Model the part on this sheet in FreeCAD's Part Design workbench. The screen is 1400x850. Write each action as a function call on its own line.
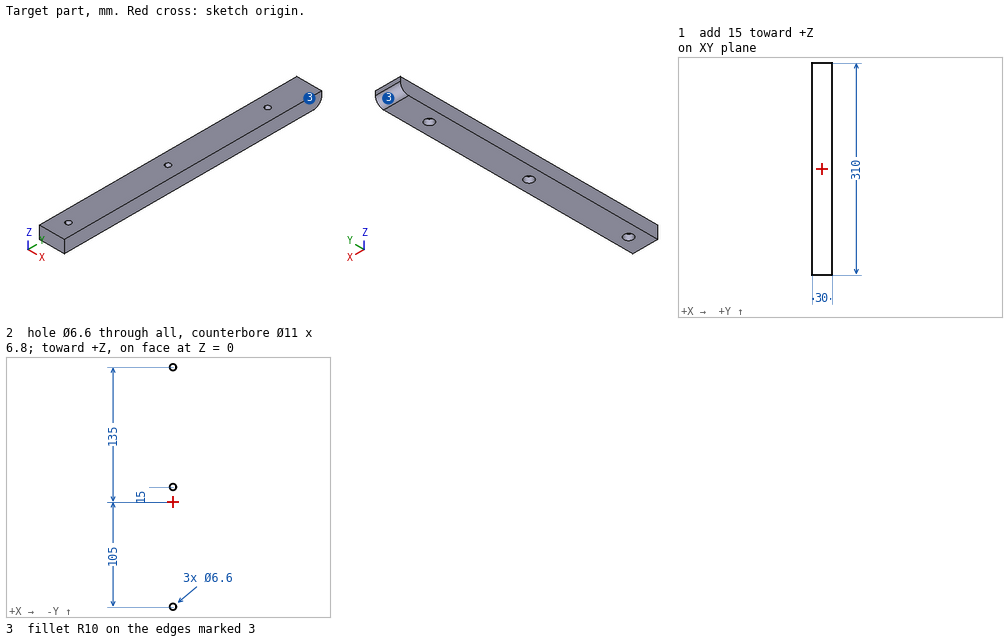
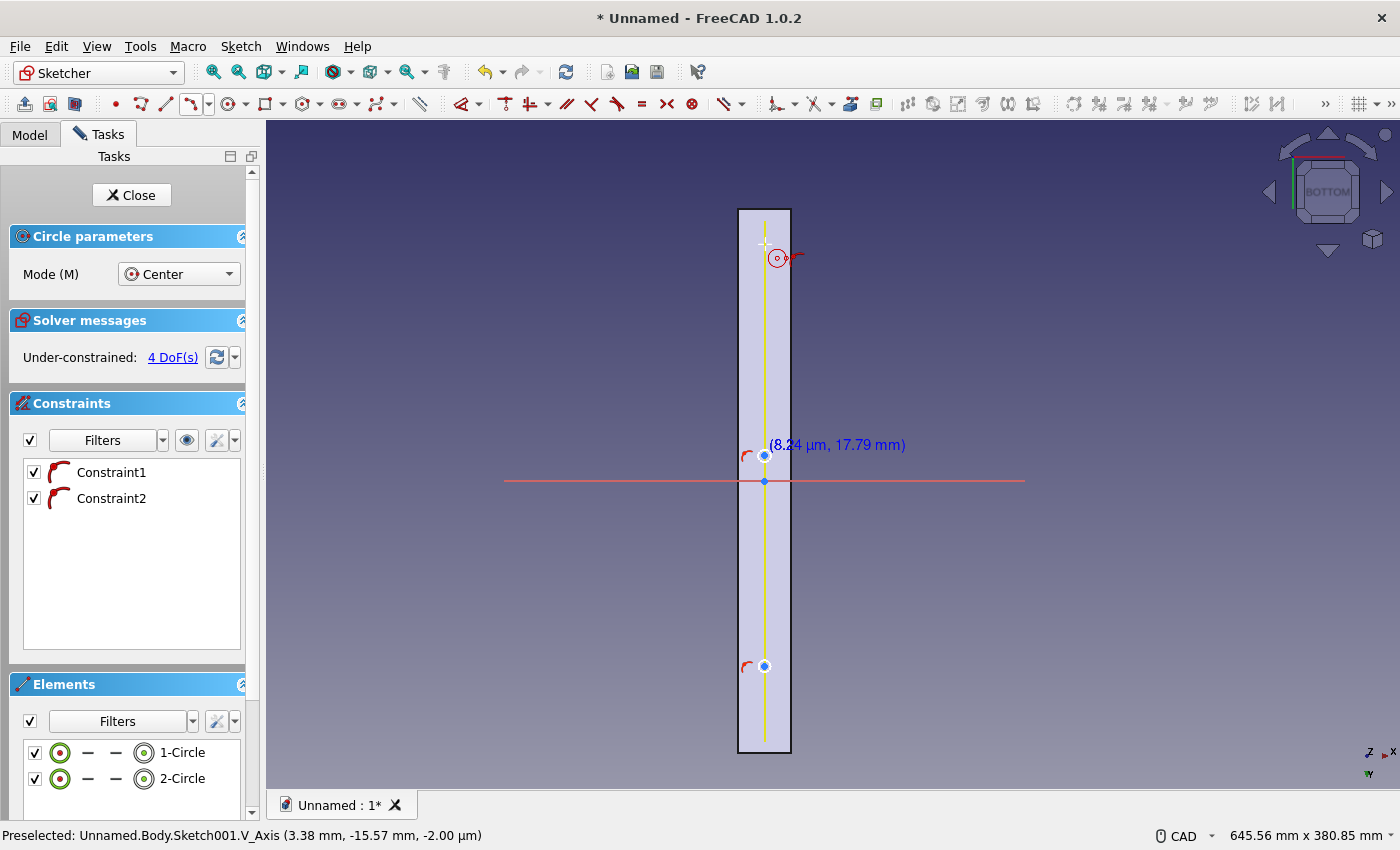
click(765, 244)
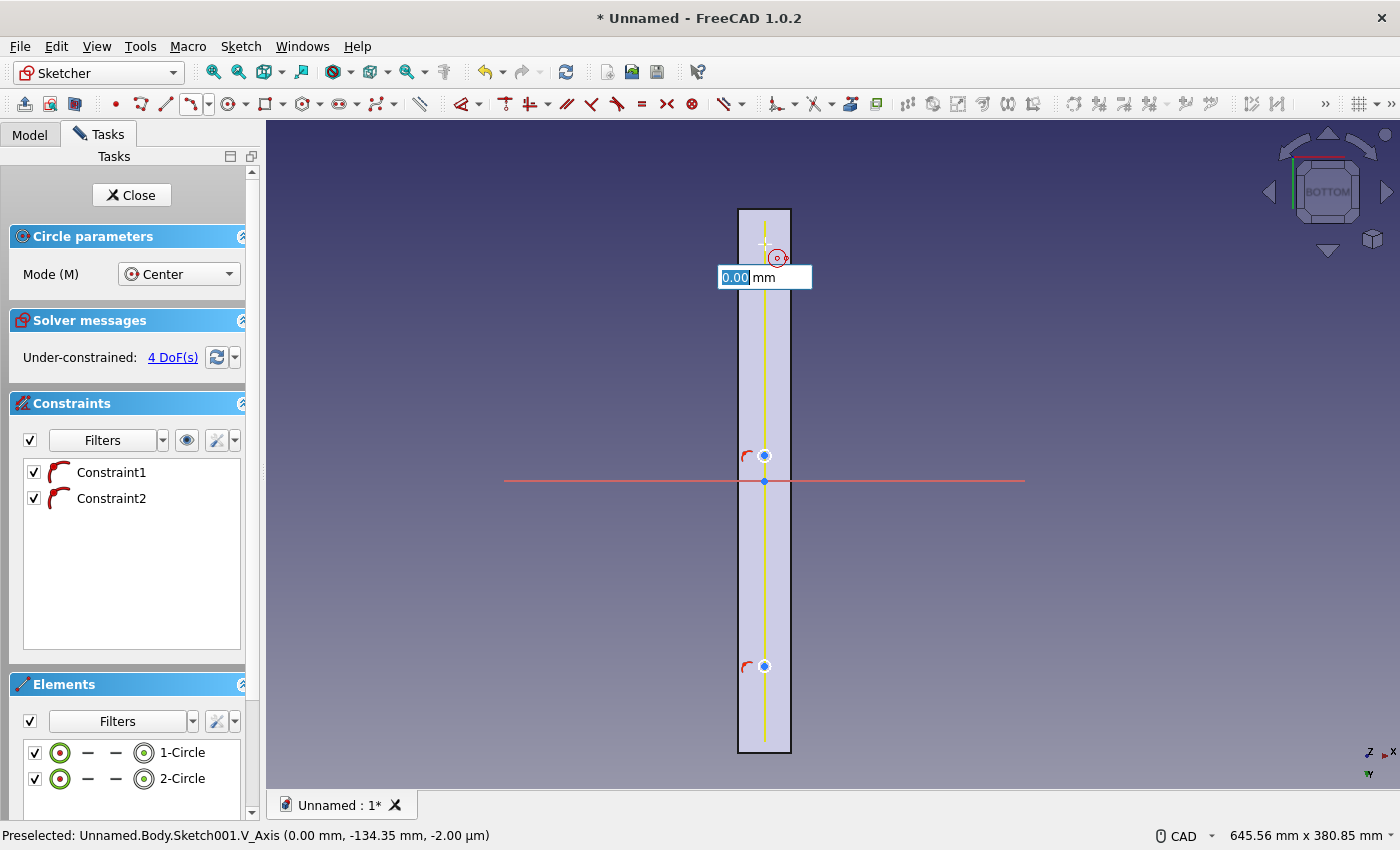
scroll(770, 242, up, 6)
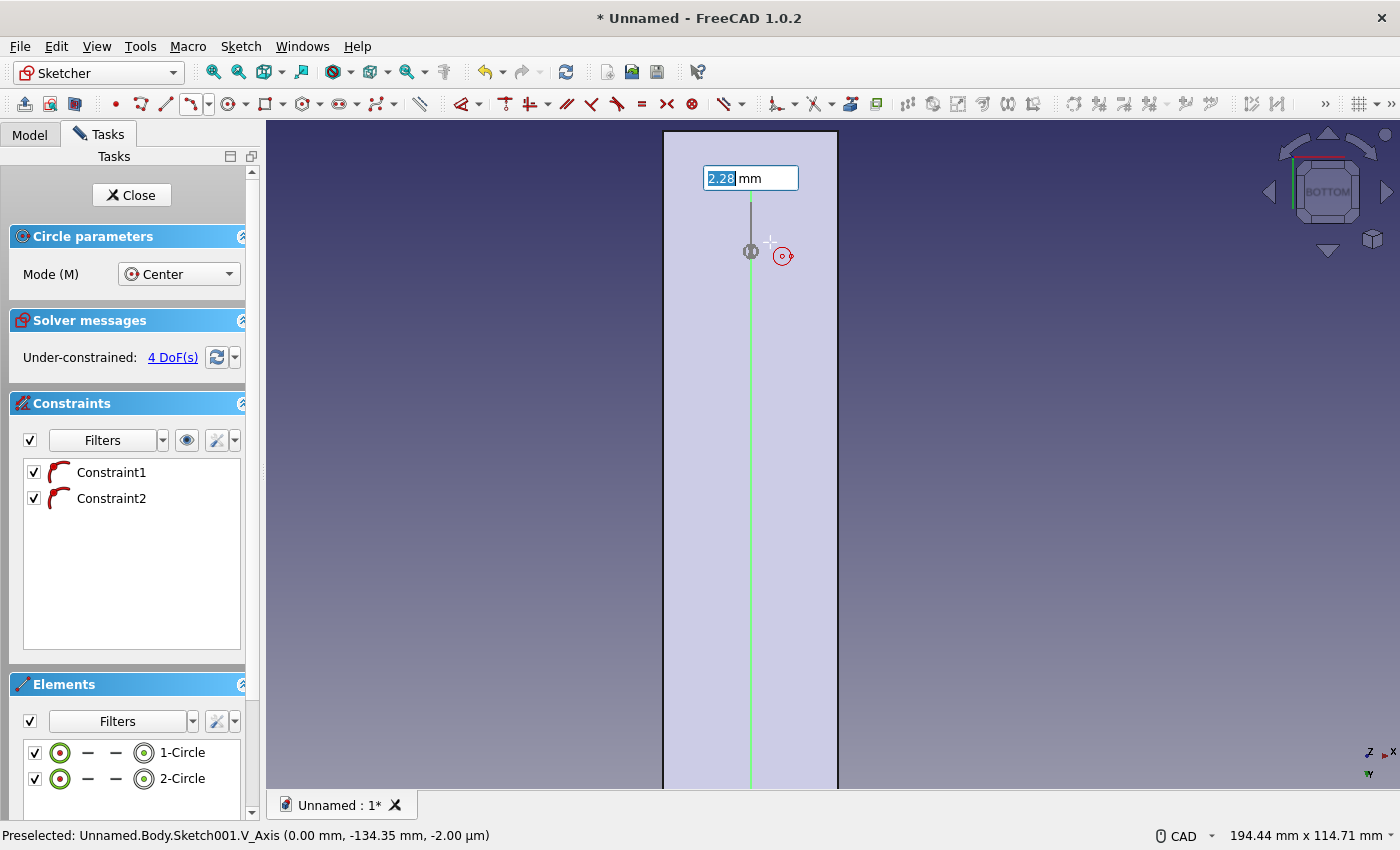
click(769, 241)
key(Escape)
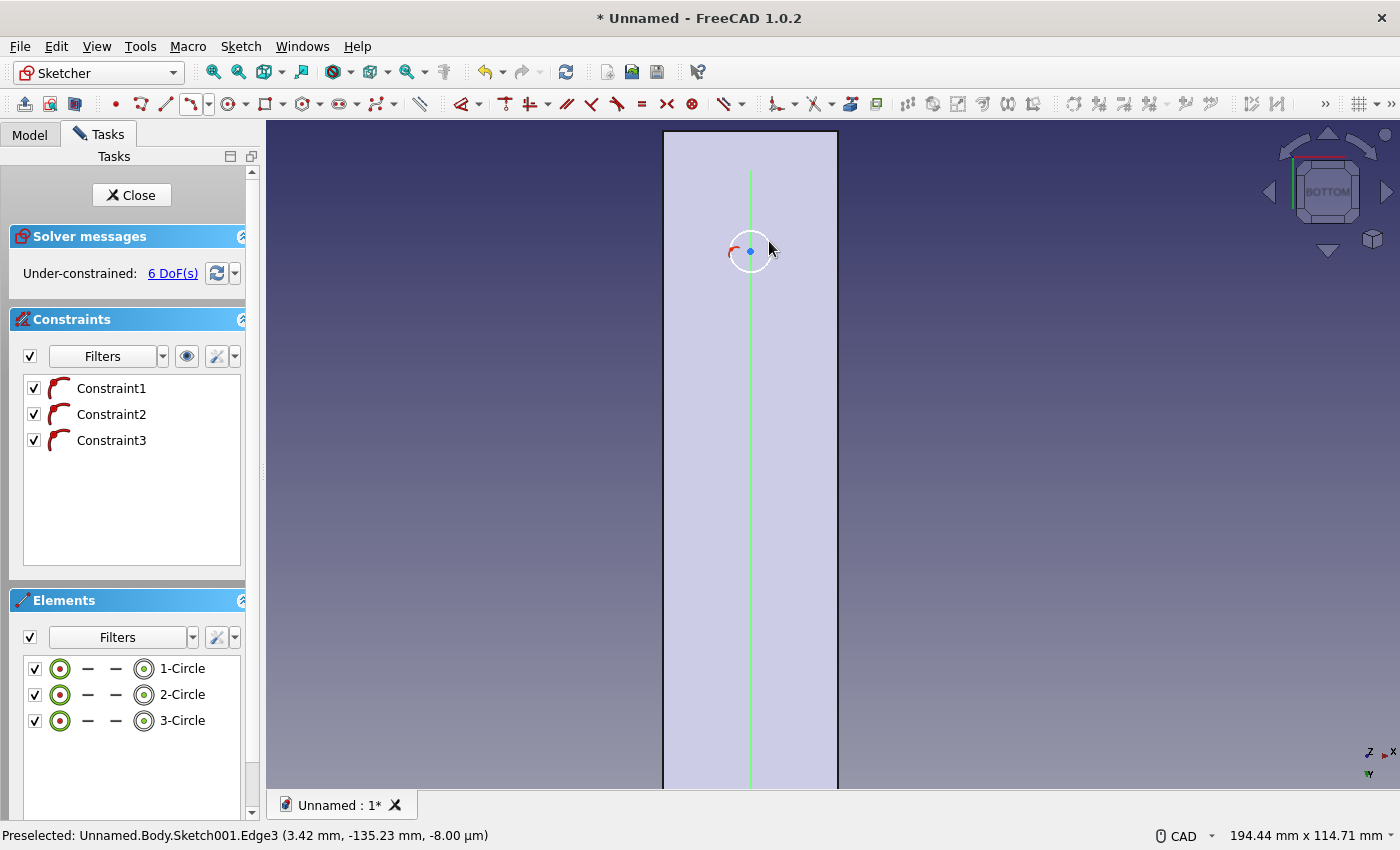
scroll(770, 242, down, 6)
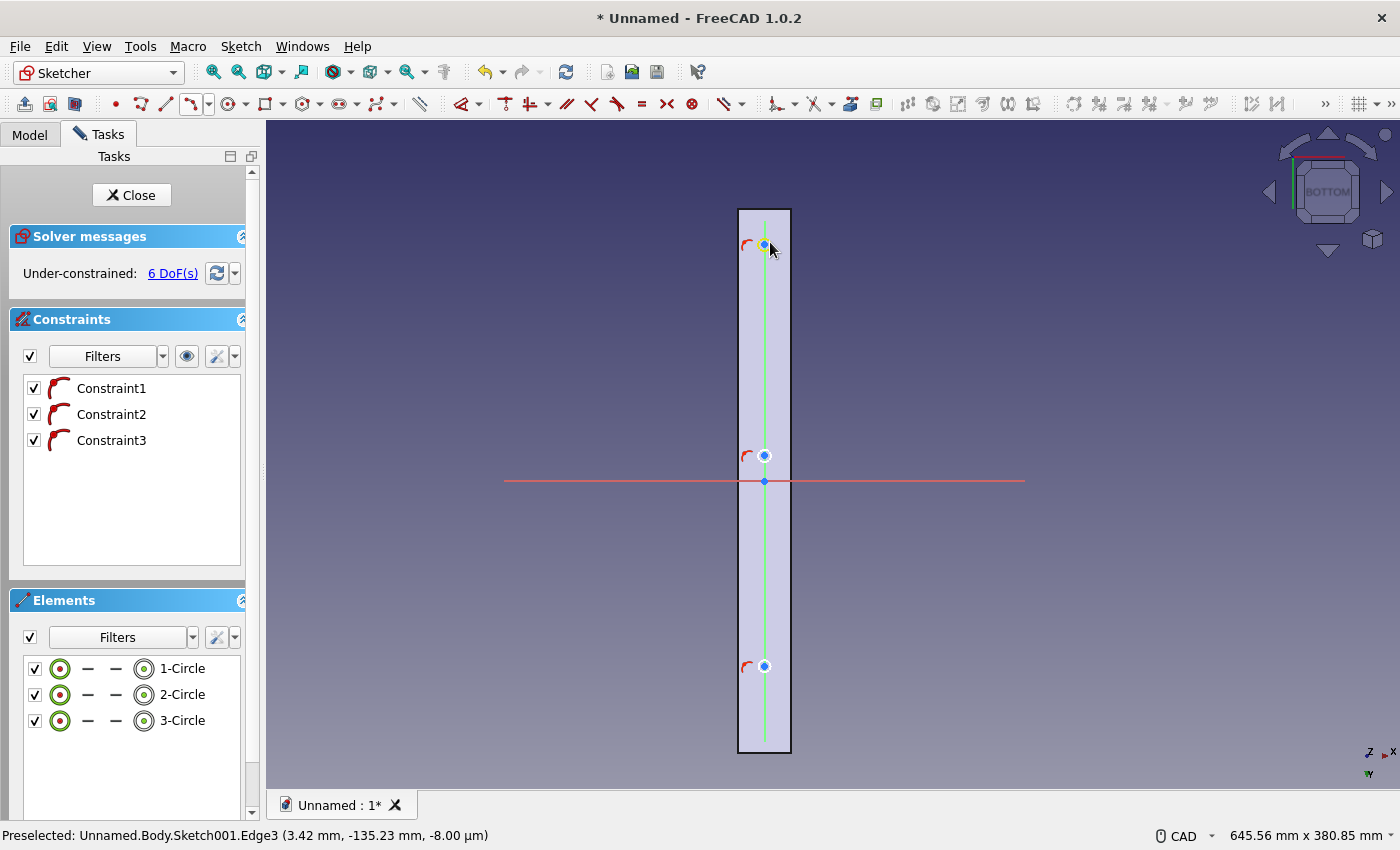
scroll(769, 662, up, 6)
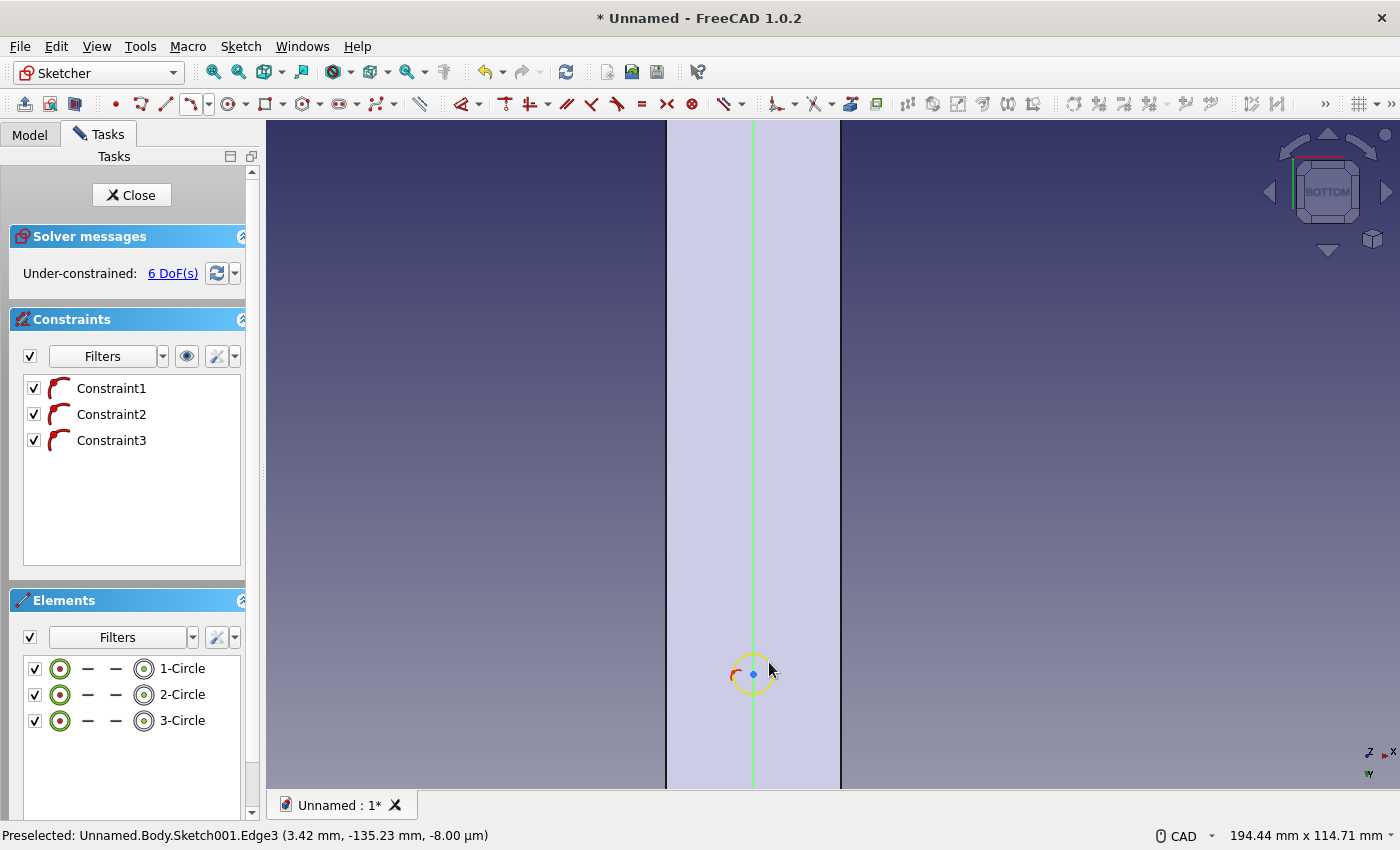
click(767, 660)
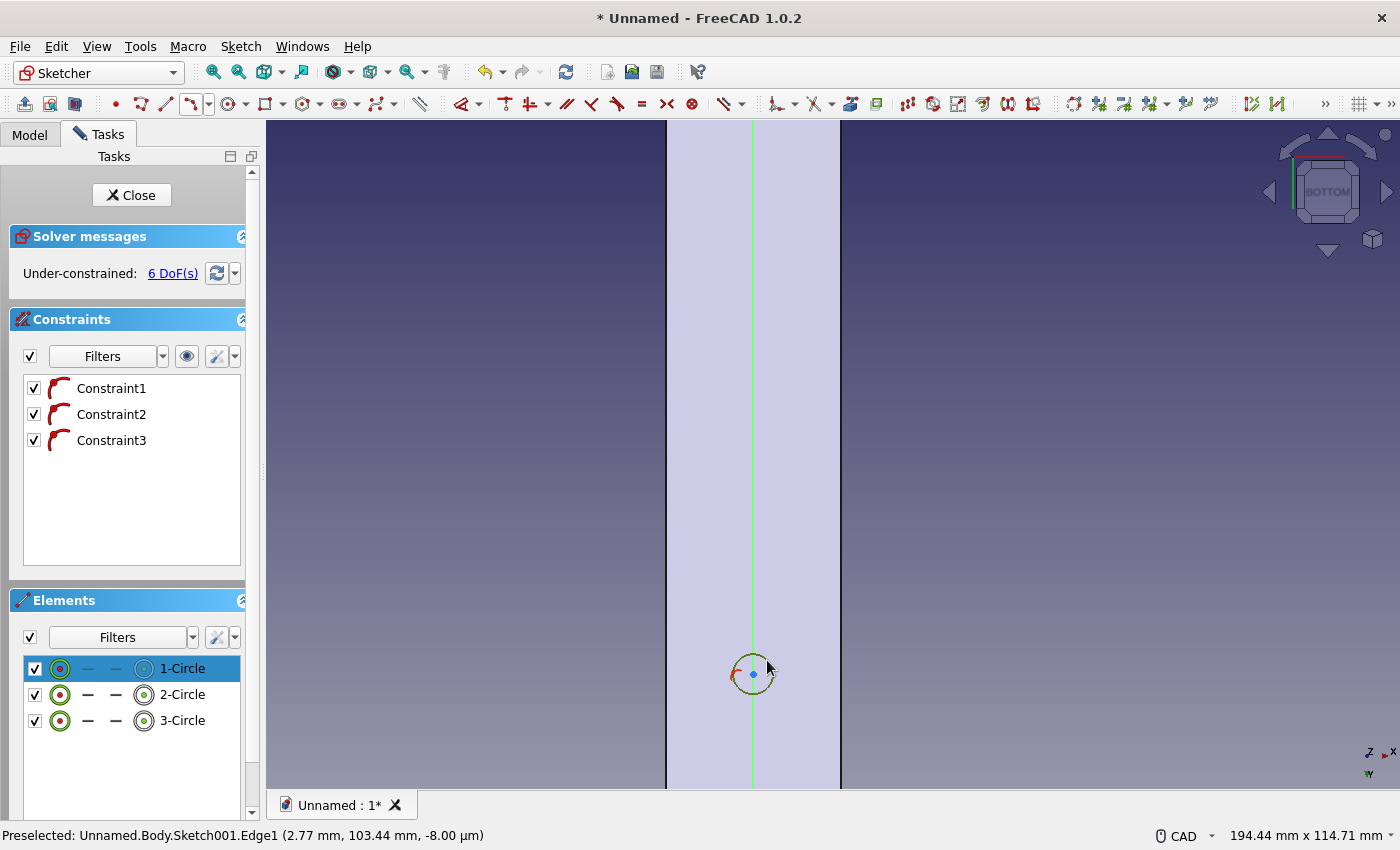
scroll(769, 663, down, 6)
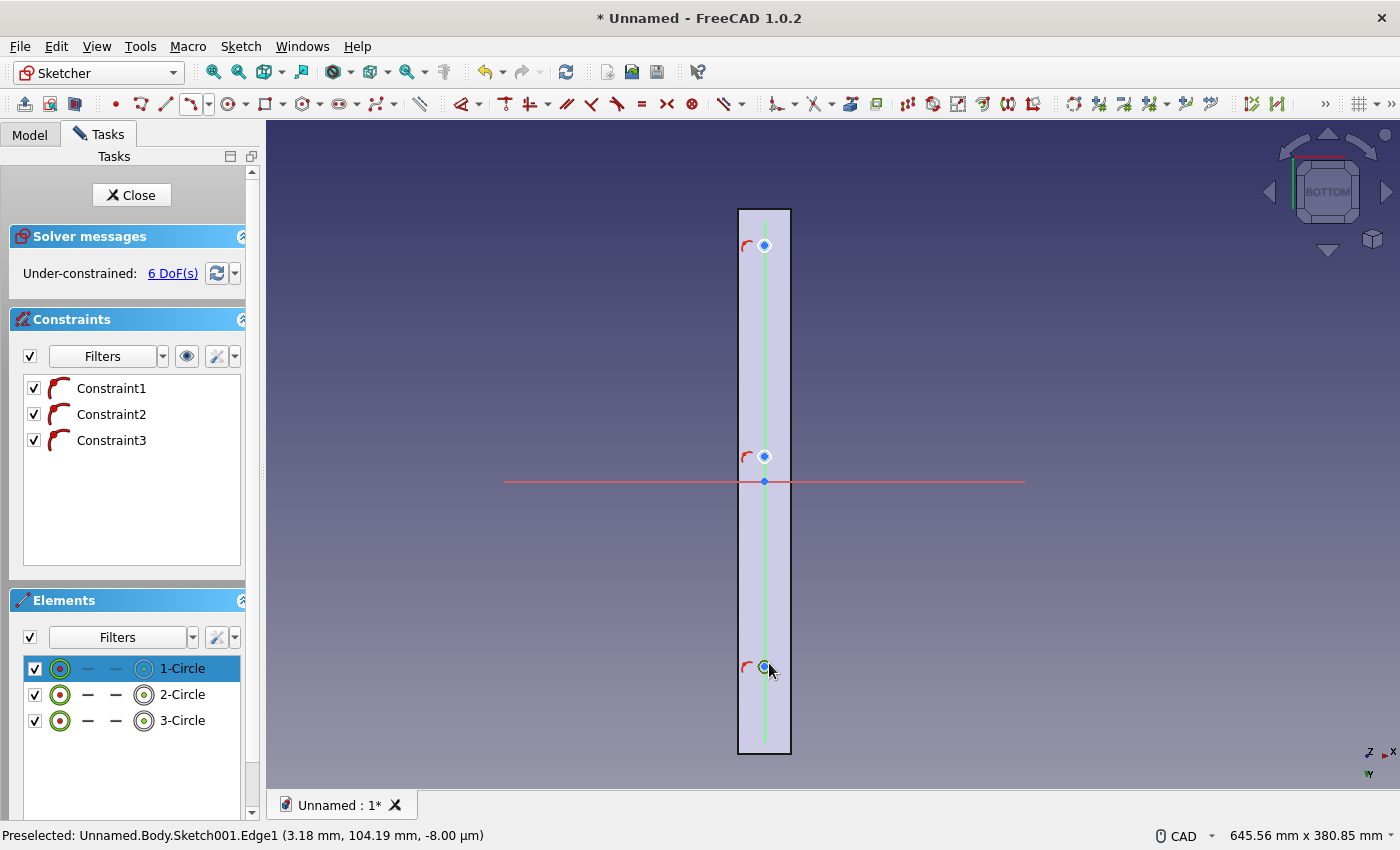
scroll(769, 452, up, 6)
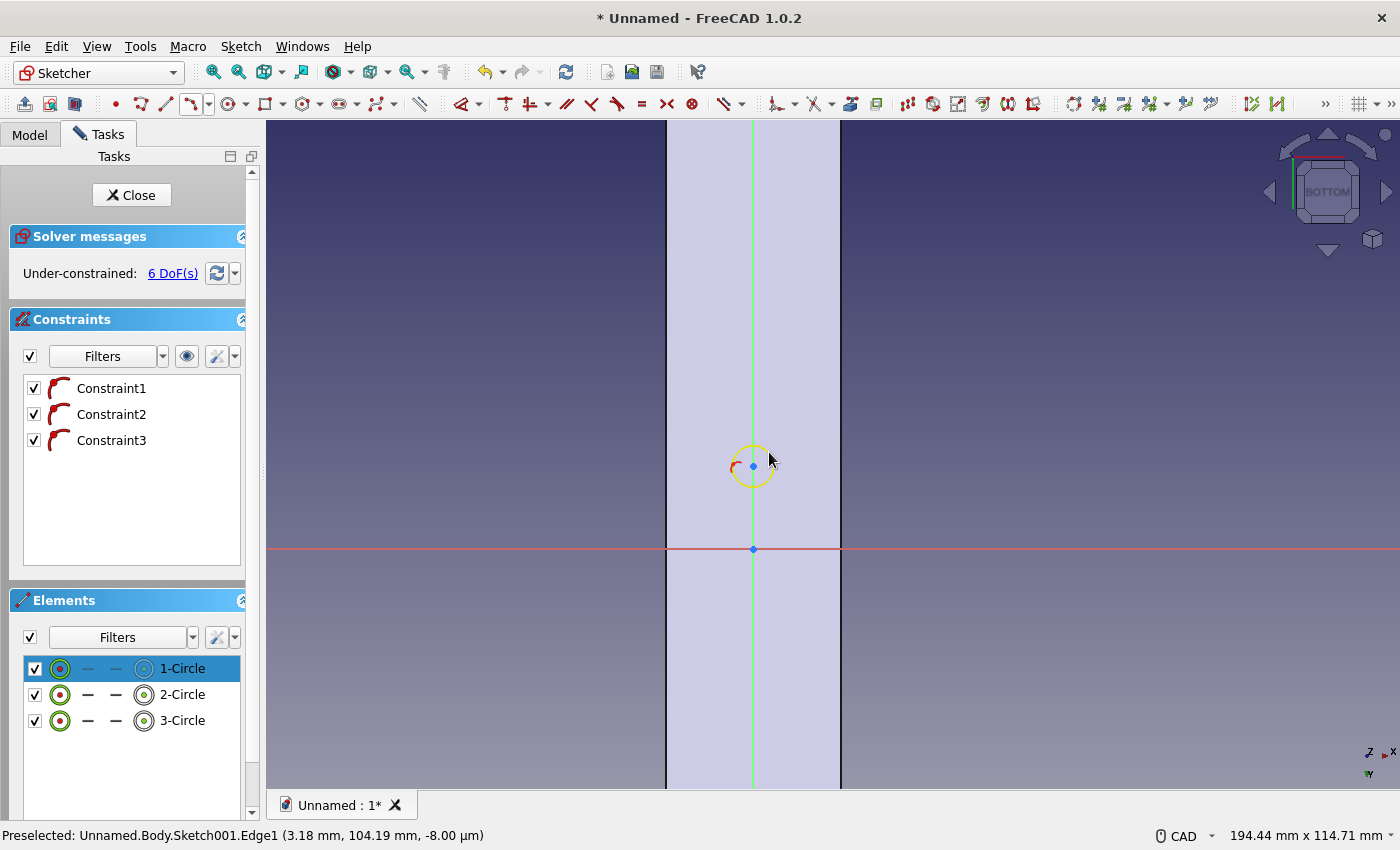
click(768, 452)